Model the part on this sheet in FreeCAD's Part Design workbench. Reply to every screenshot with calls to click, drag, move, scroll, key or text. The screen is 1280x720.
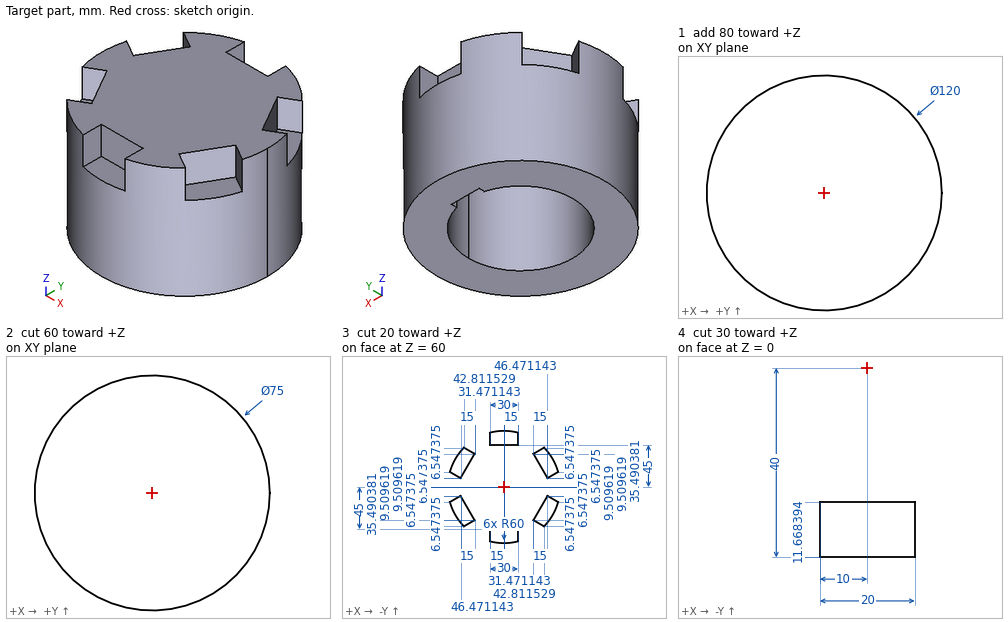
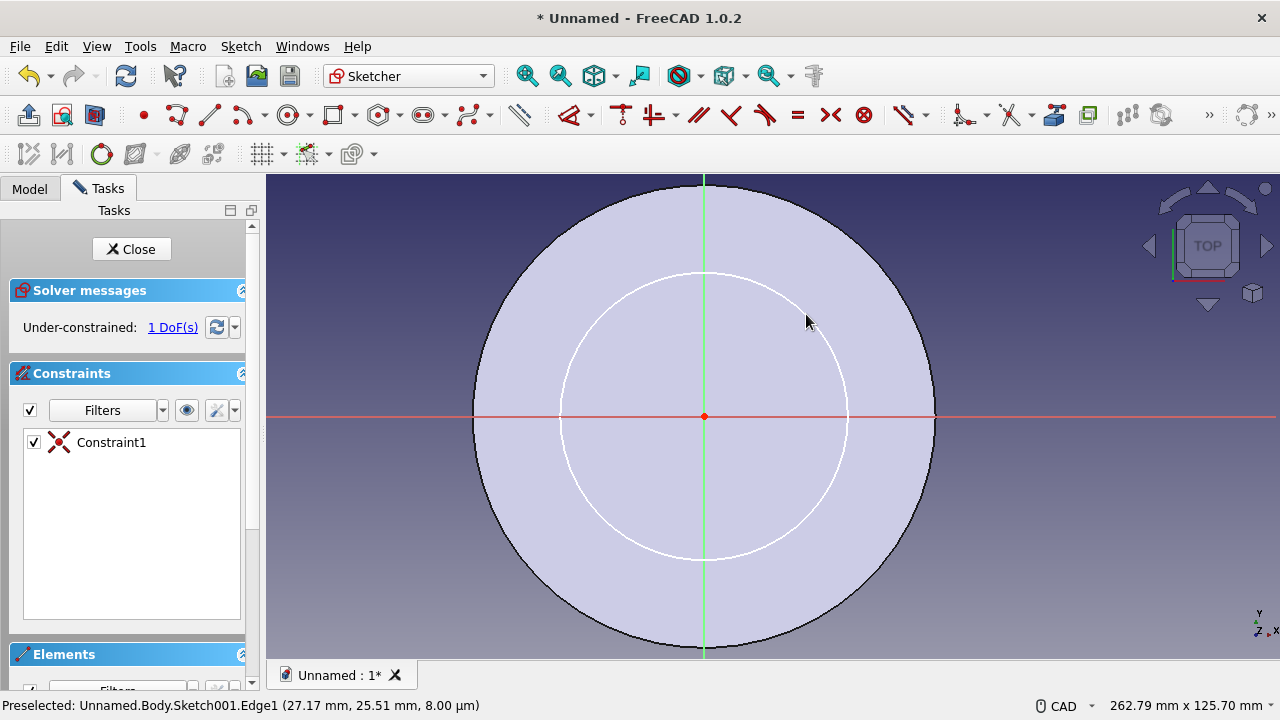
click(568, 116)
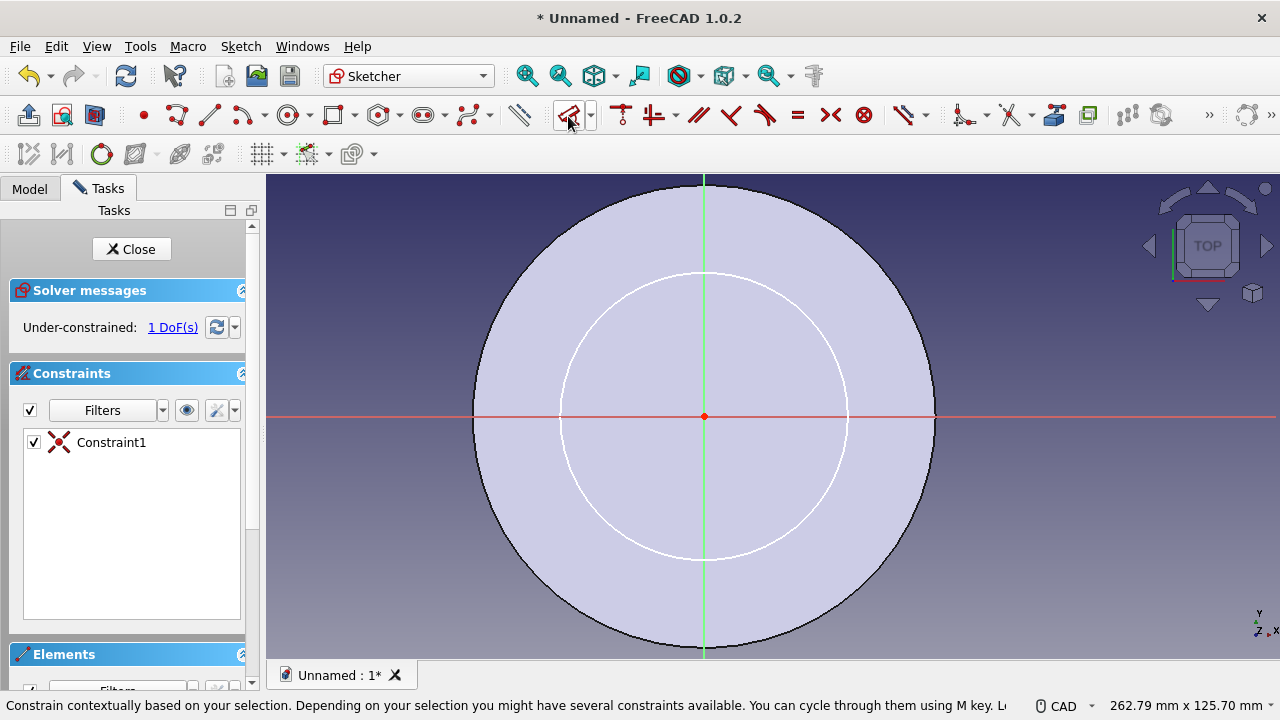
click(805, 314)
click(827, 291)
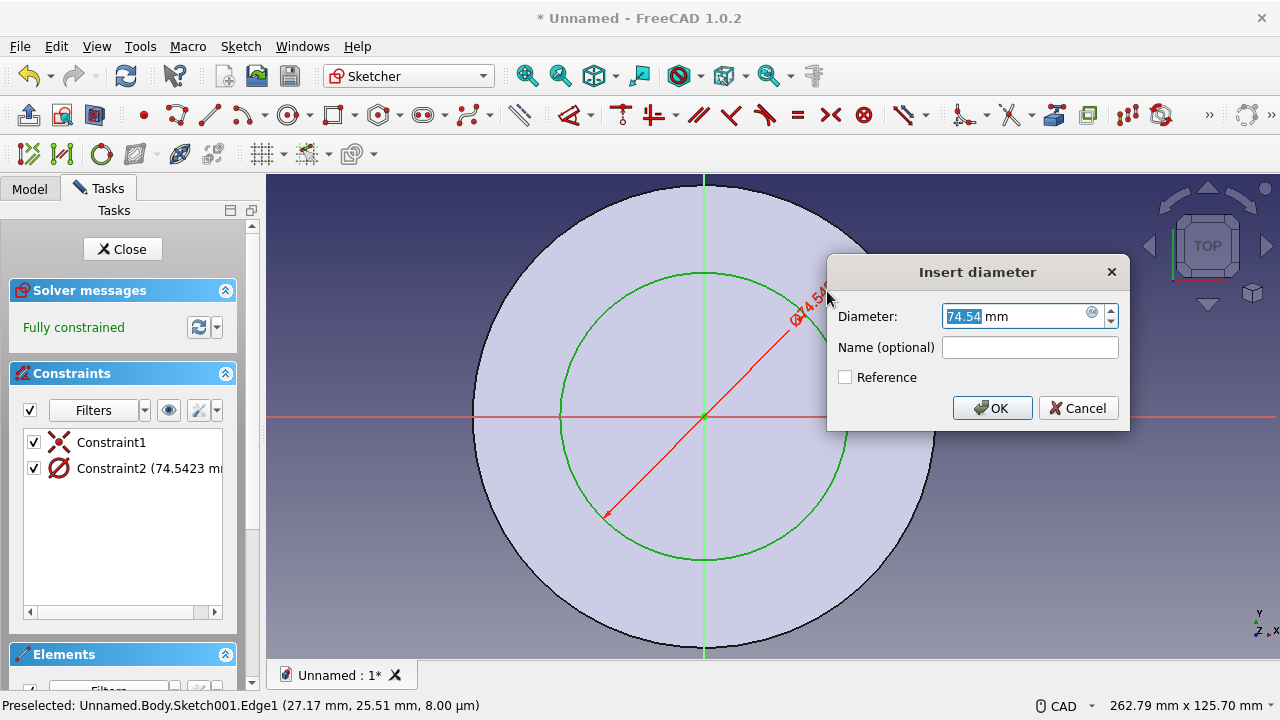
text(75)
key(Return)
key(Escape)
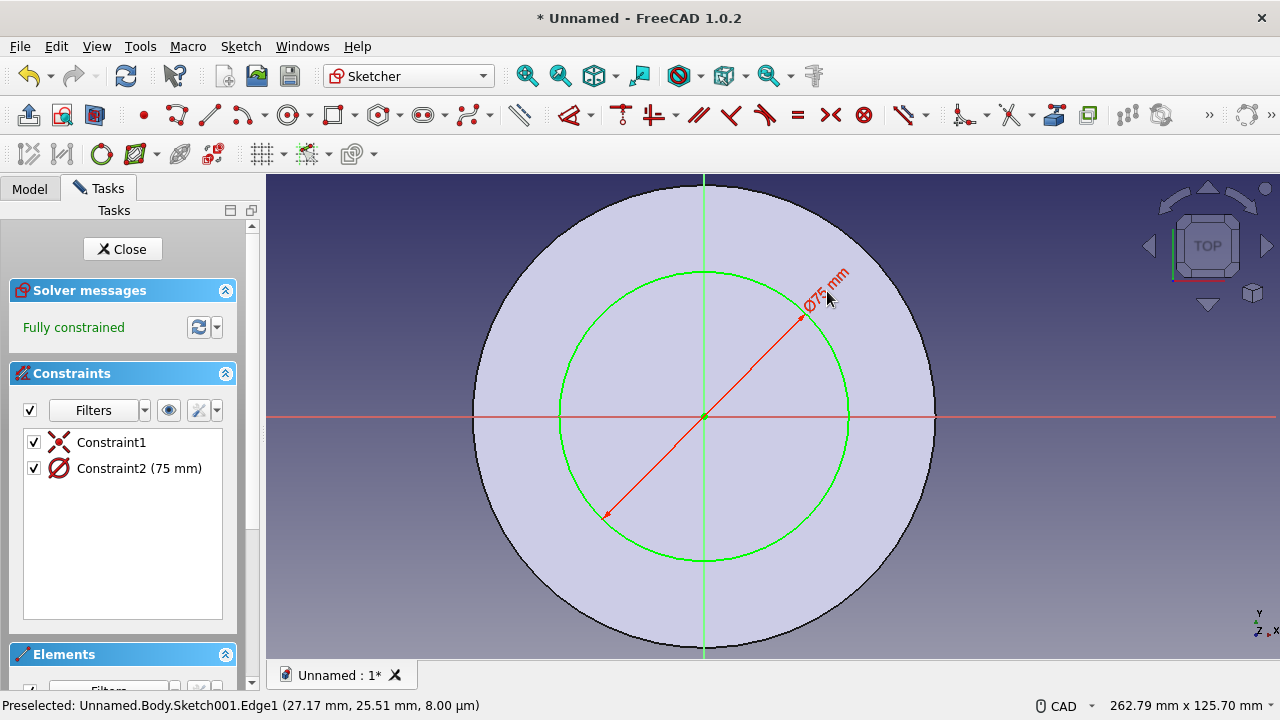
click(123, 249)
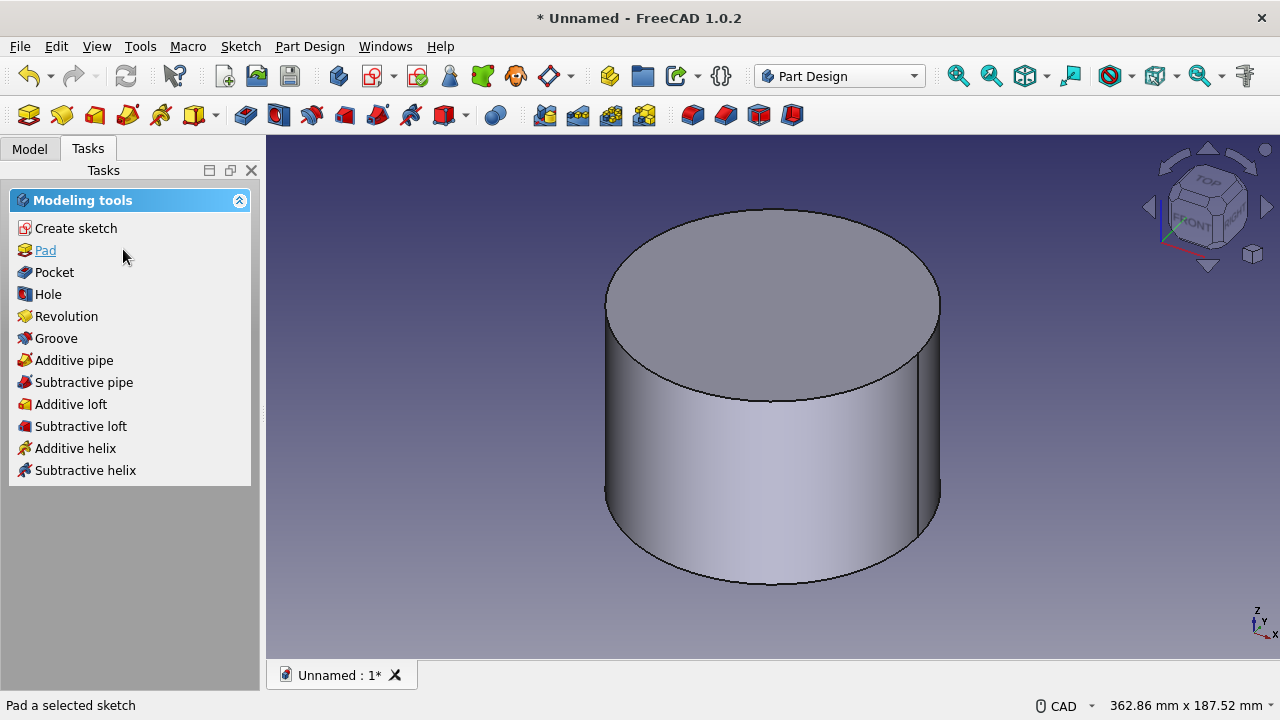
click(246, 116)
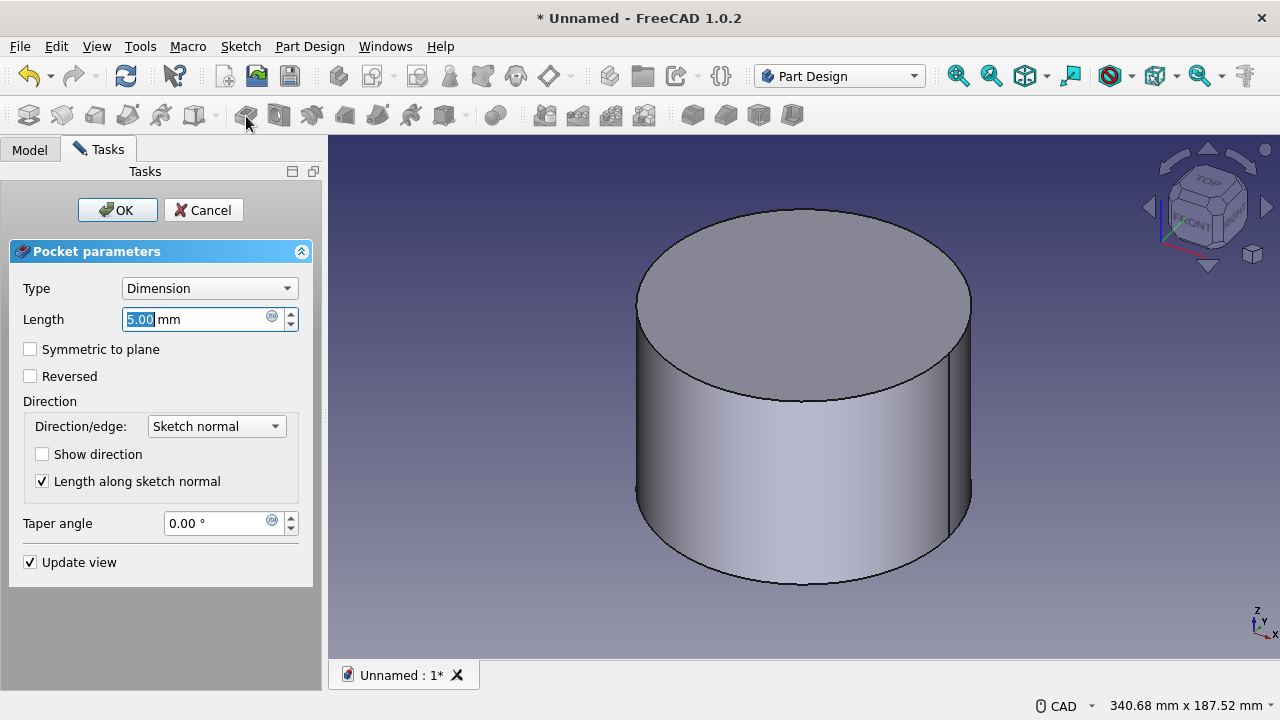
text(60)
key(Tab)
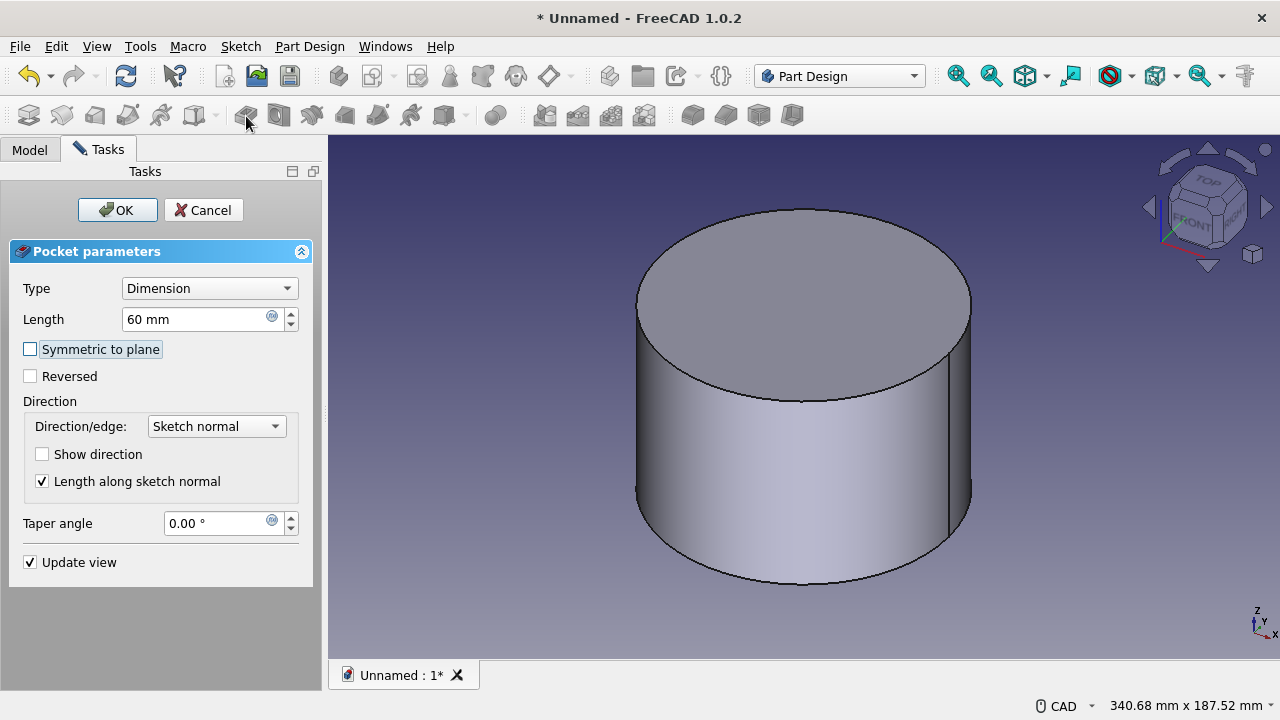
click(31, 376)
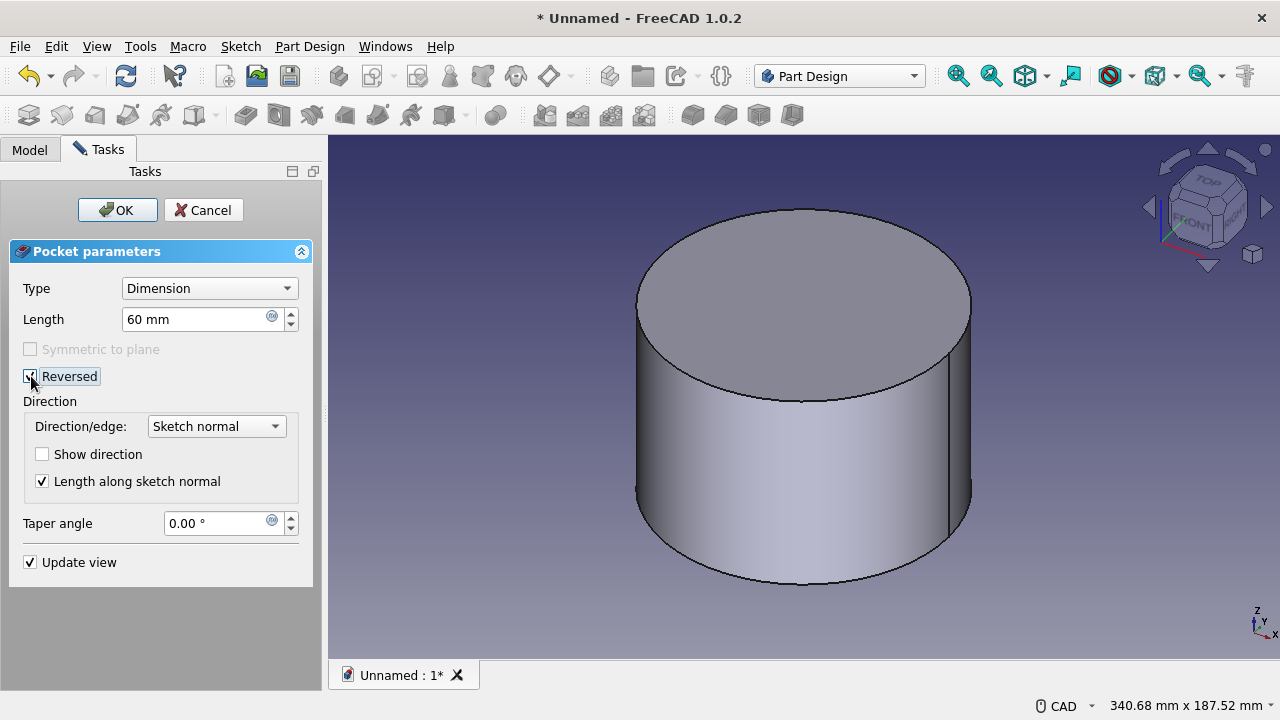
click(118, 210)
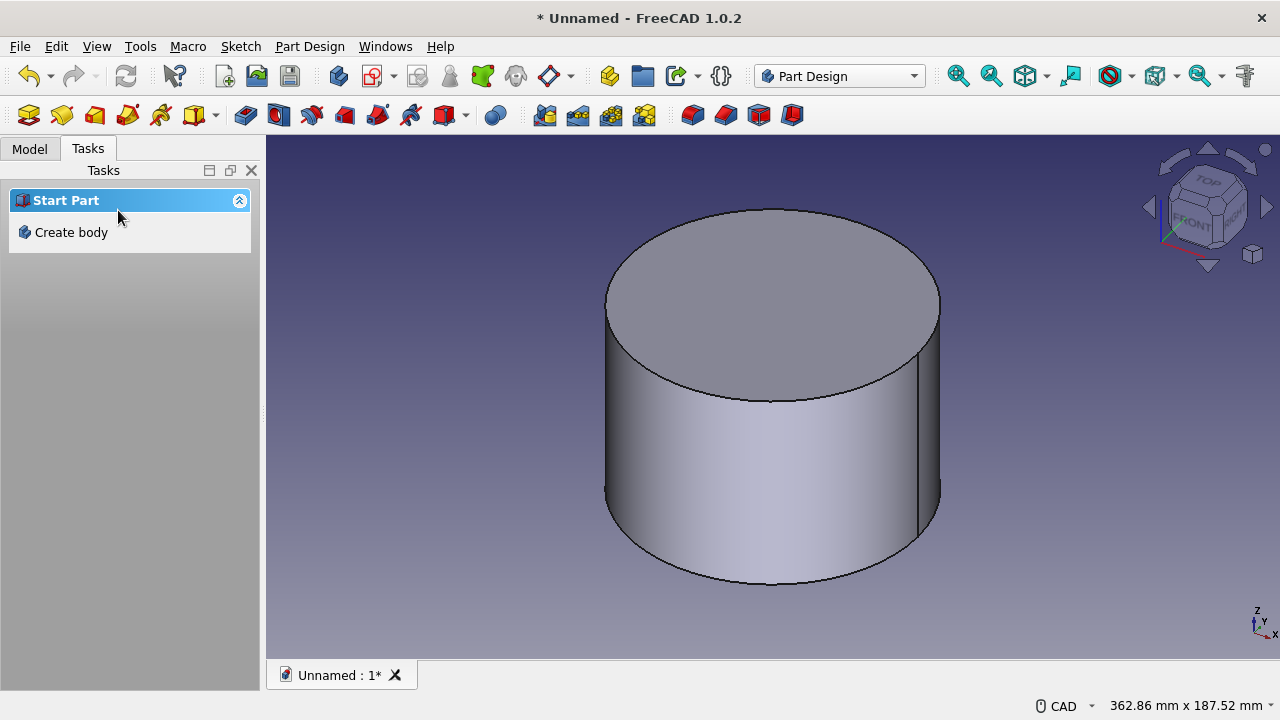
key(5)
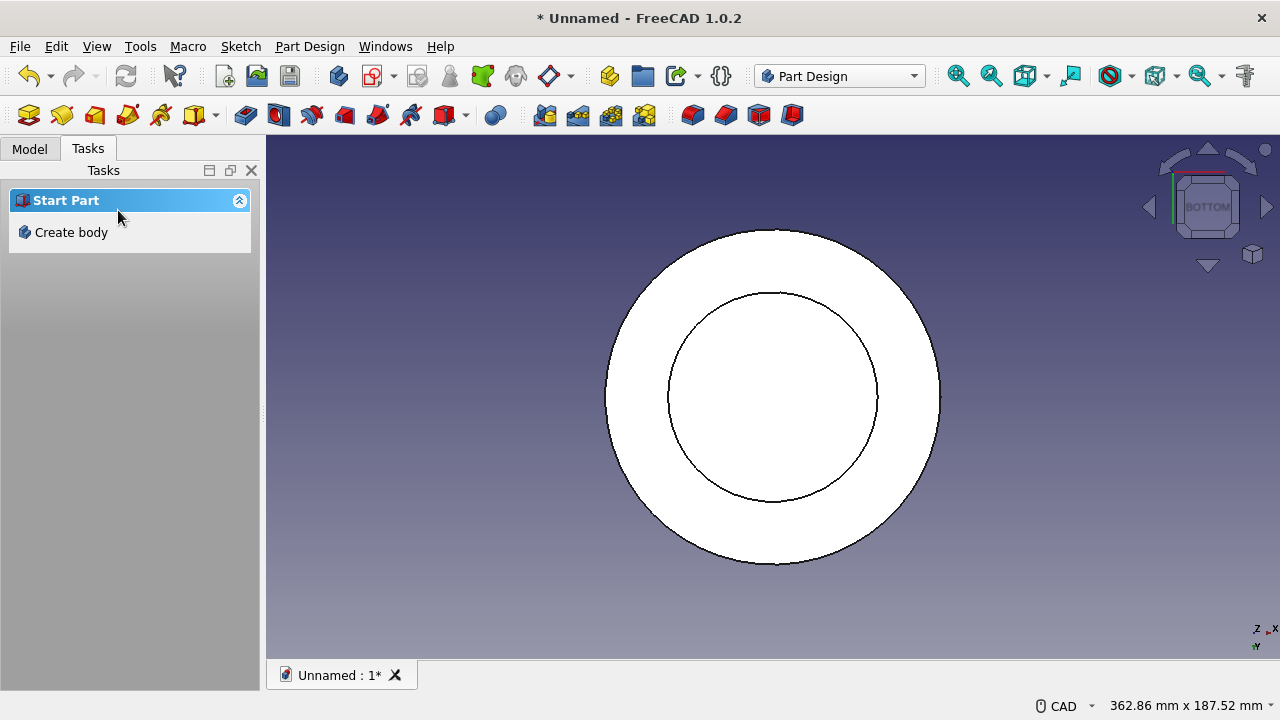
click(773, 396)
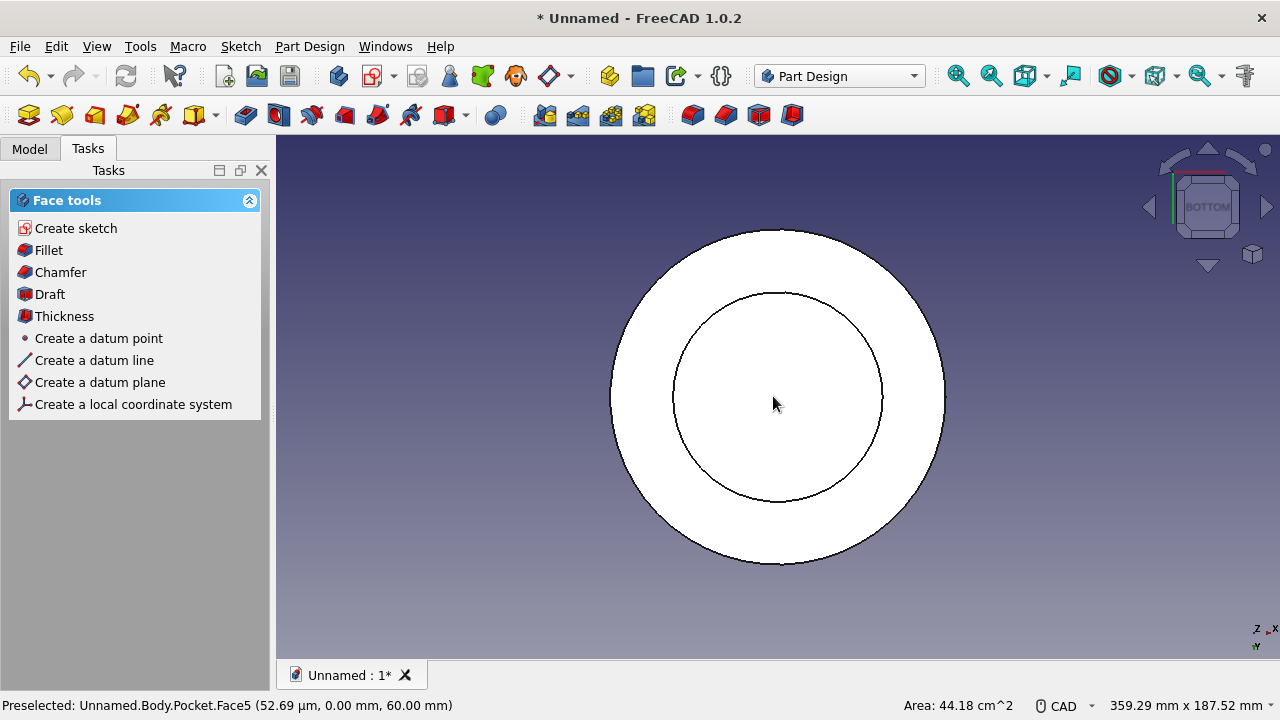
click(372, 76)